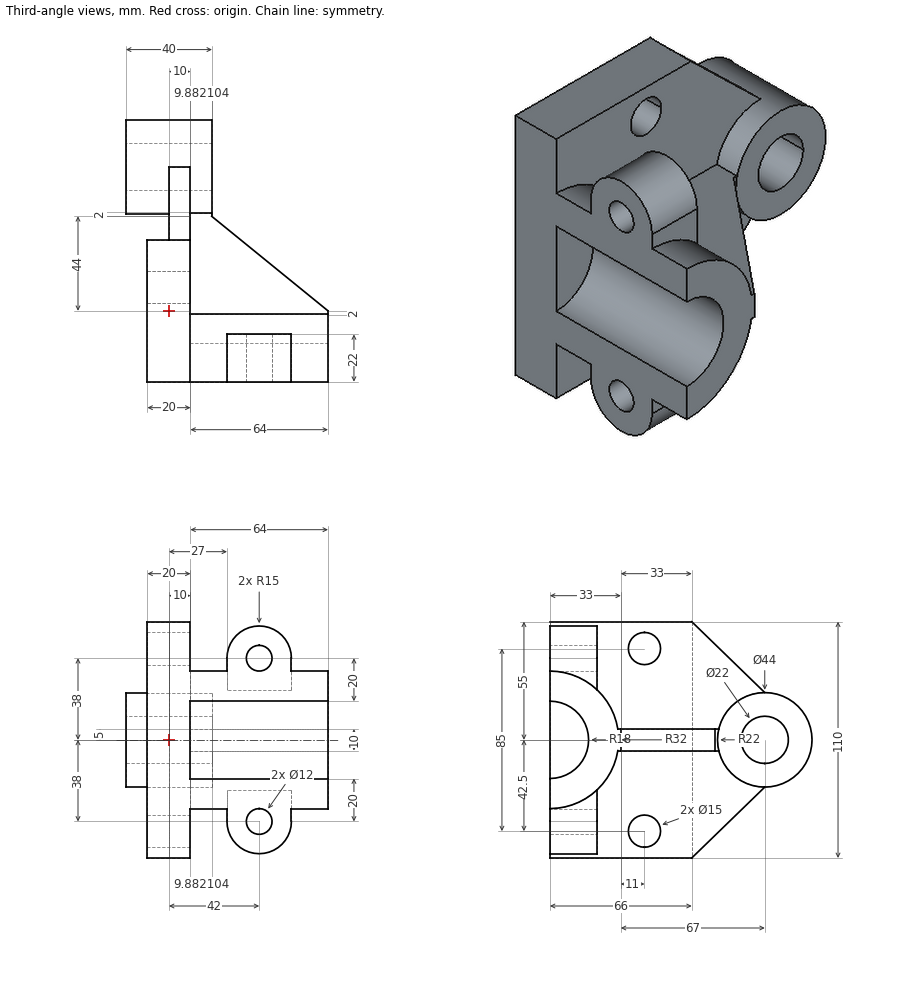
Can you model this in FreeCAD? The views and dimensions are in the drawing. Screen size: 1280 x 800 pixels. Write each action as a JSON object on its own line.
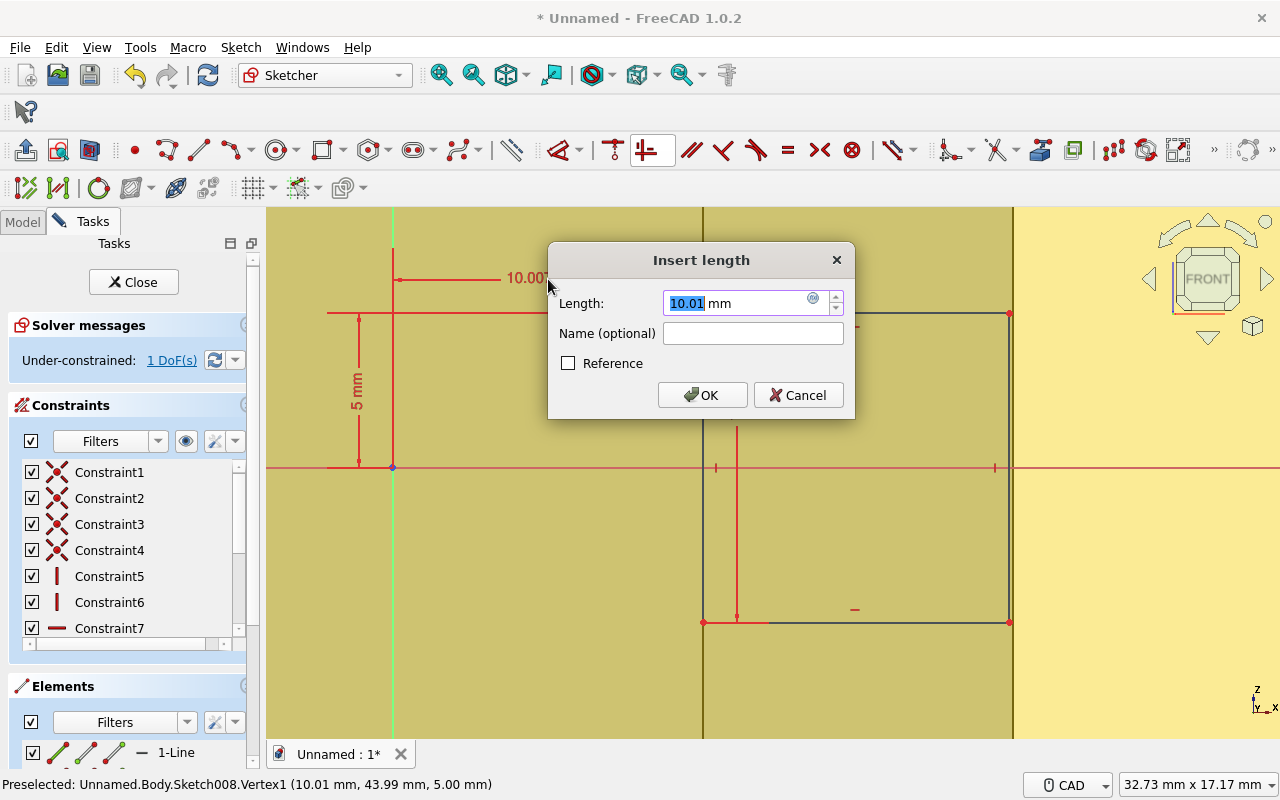
{"action": "type", "text": "10"}
{"action": "key", "text": "Return"}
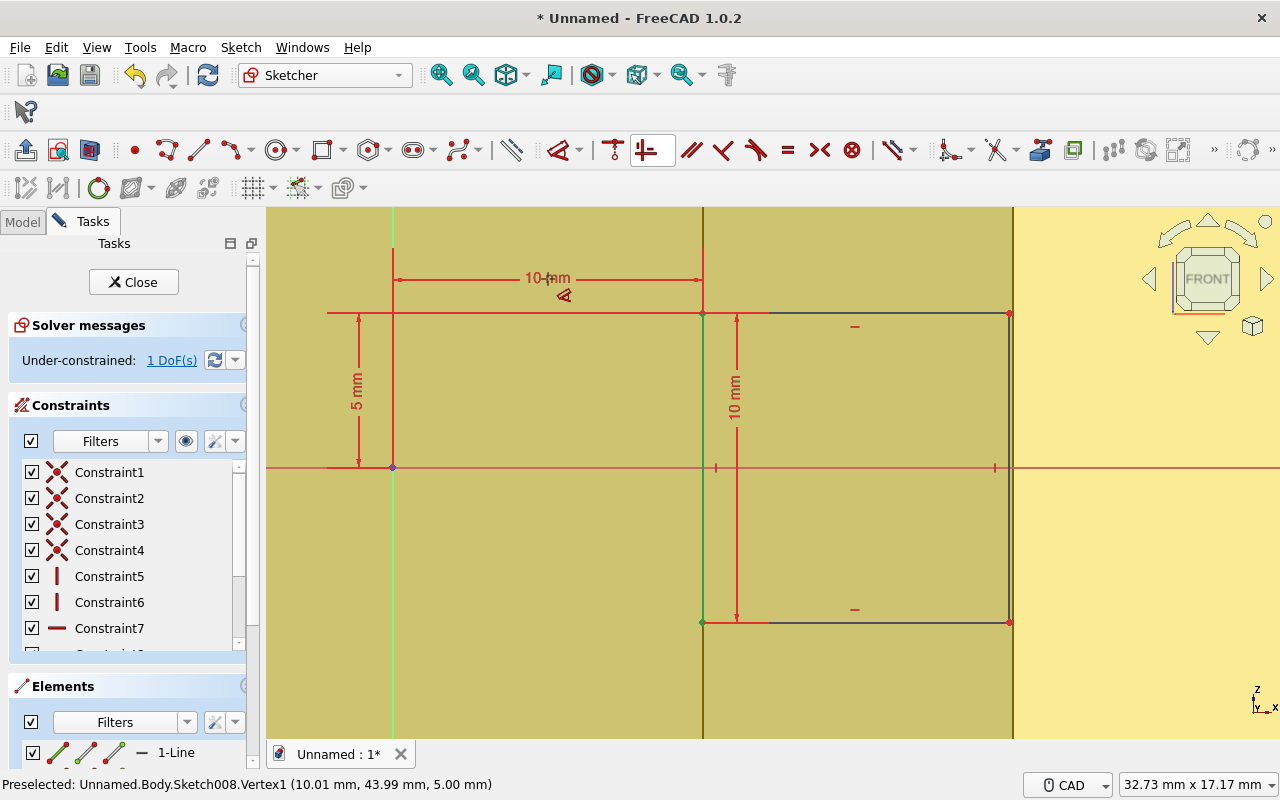
{"action": "left_click", "coordinate": [795, 623]}
{"action": "left_click", "coordinate": [856, 657]}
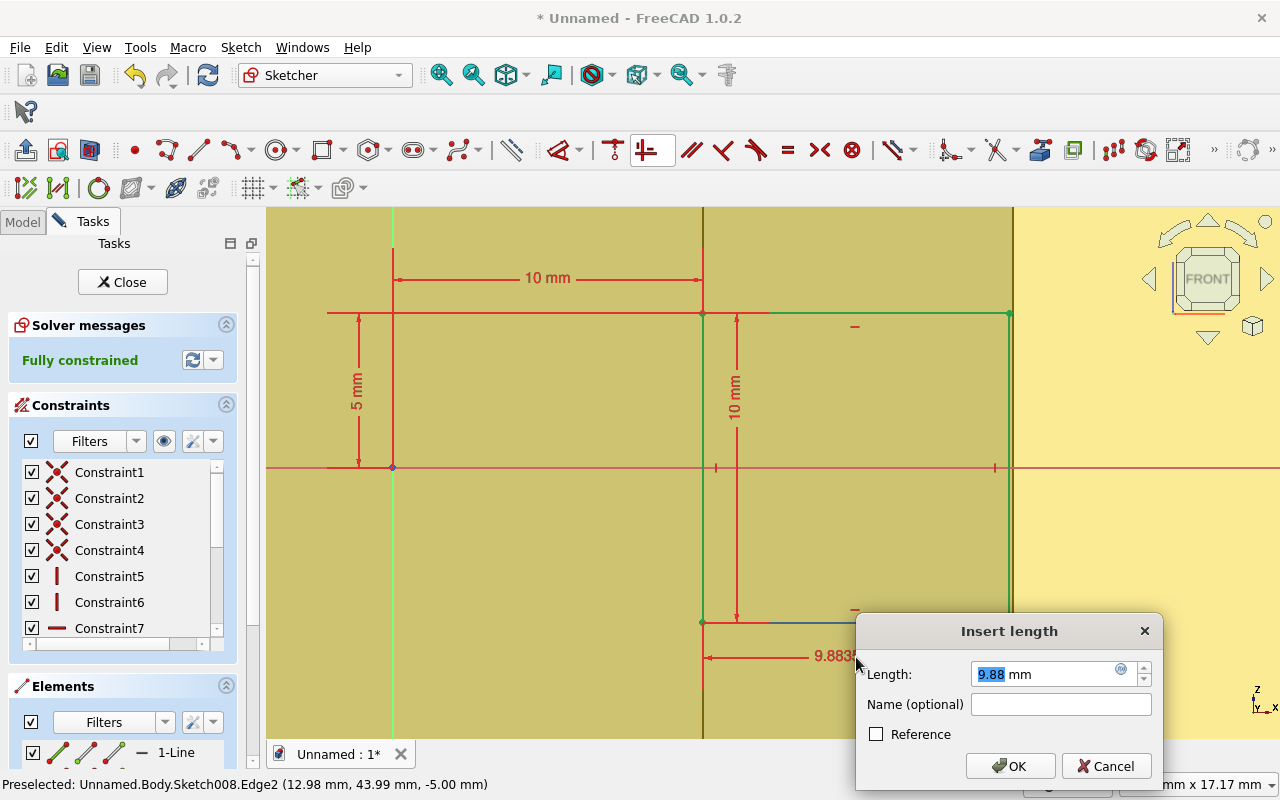
{"action": "type", "text": "9.882104"}
{"action": "key", "text": "Return"}
{"action": "key", "text": "Escape"}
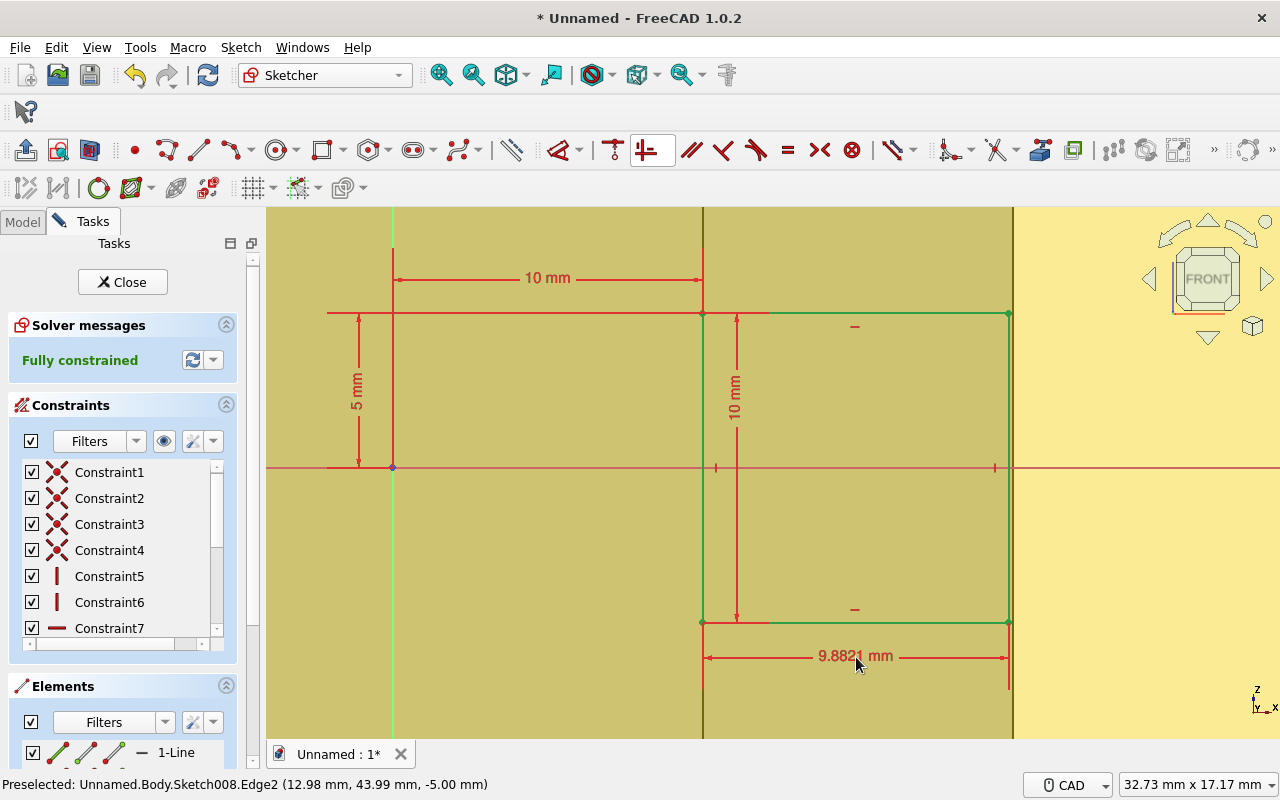
{"action": "left_click", "coordinate": [123, 282]}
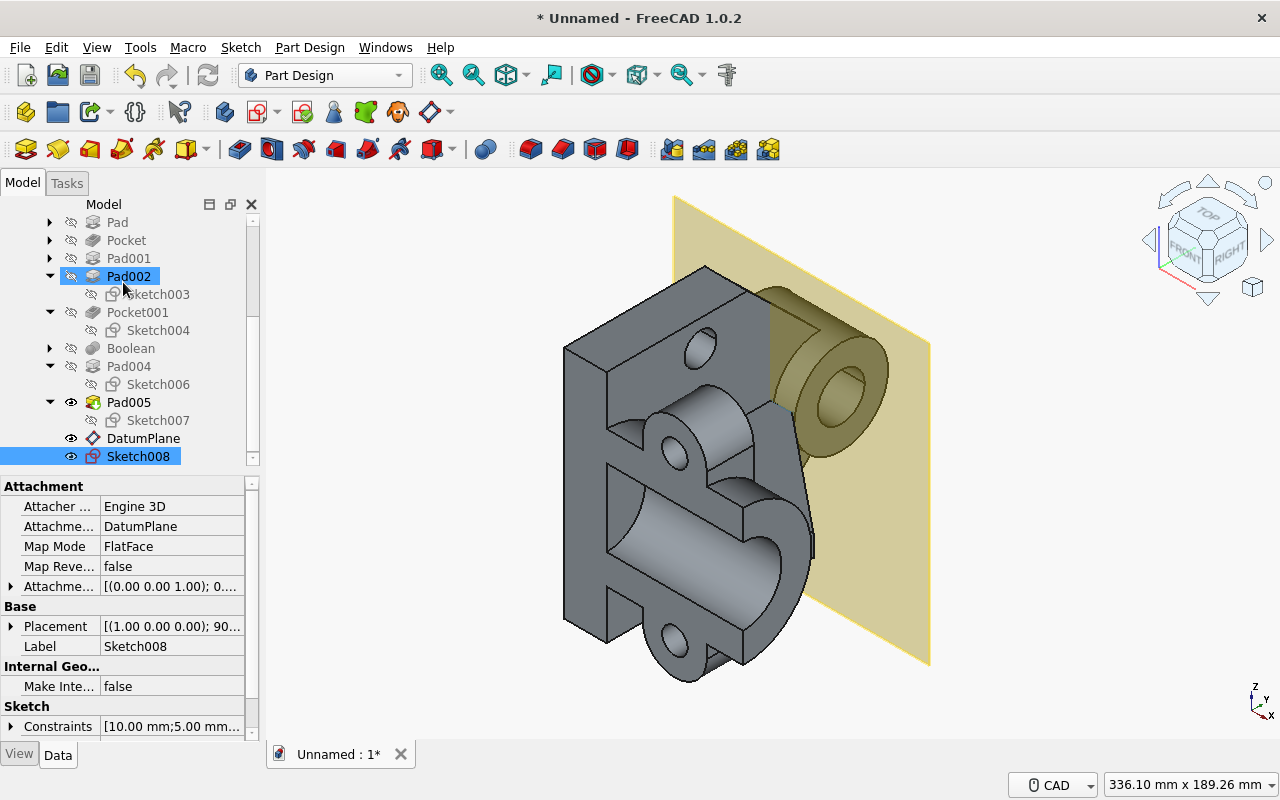
{"action": "left_click", "coordinate": [26, 150]}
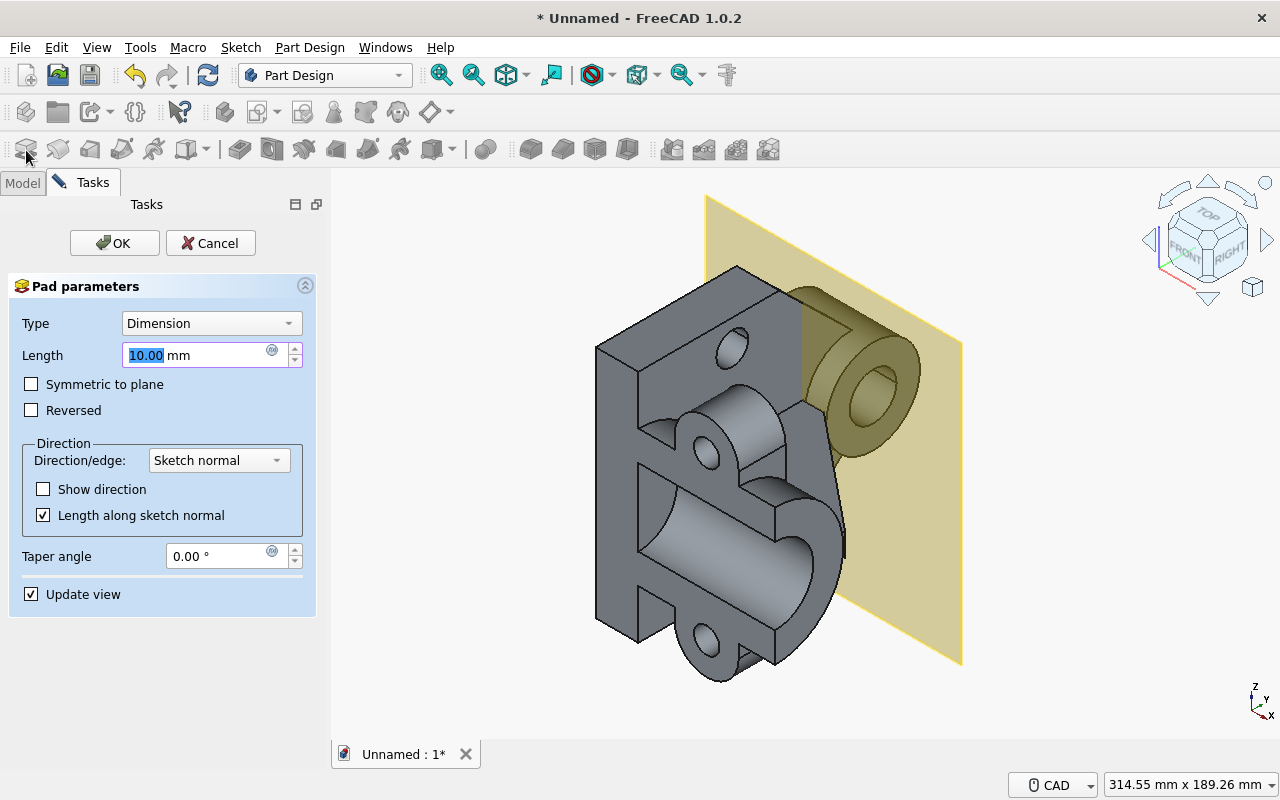
{"action": "type", "text": "2"}
{"action": "key", "text": "Tab"}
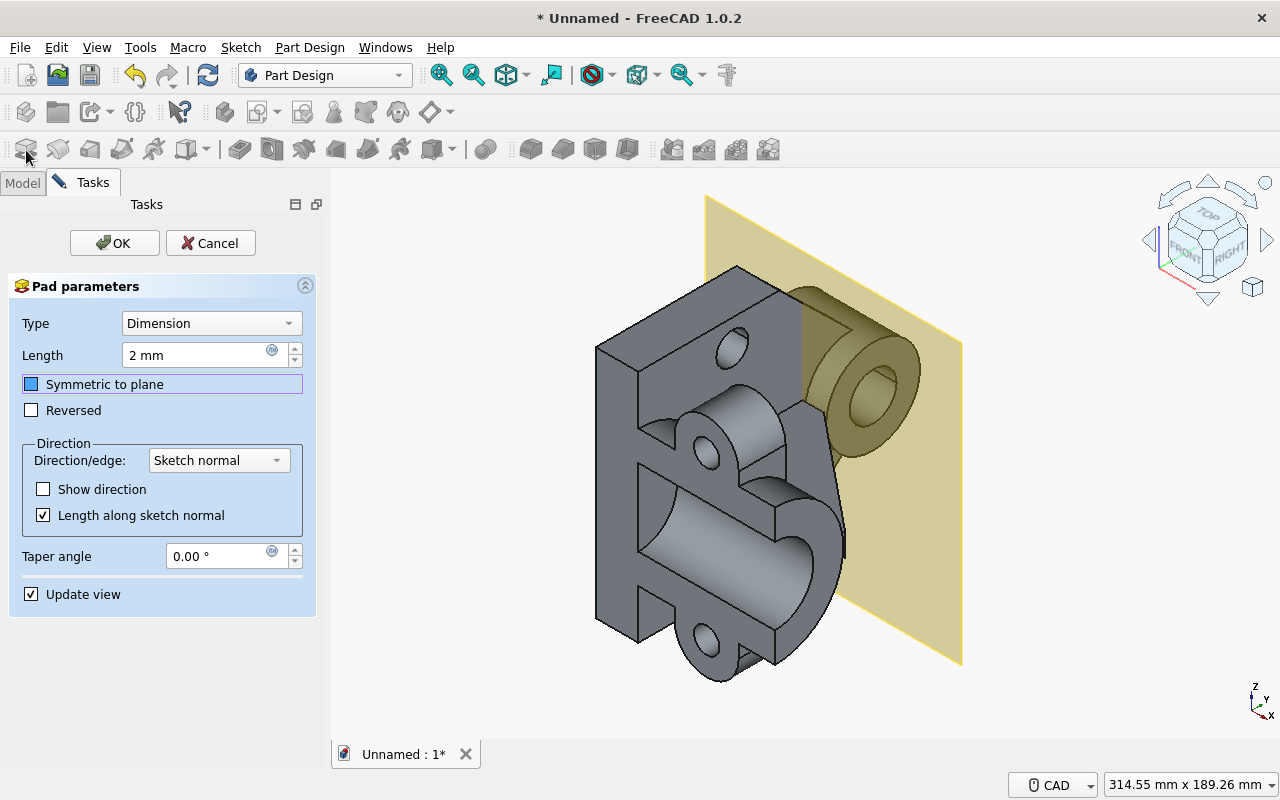
{"action": "left_click", "coordinate": [30, 410]}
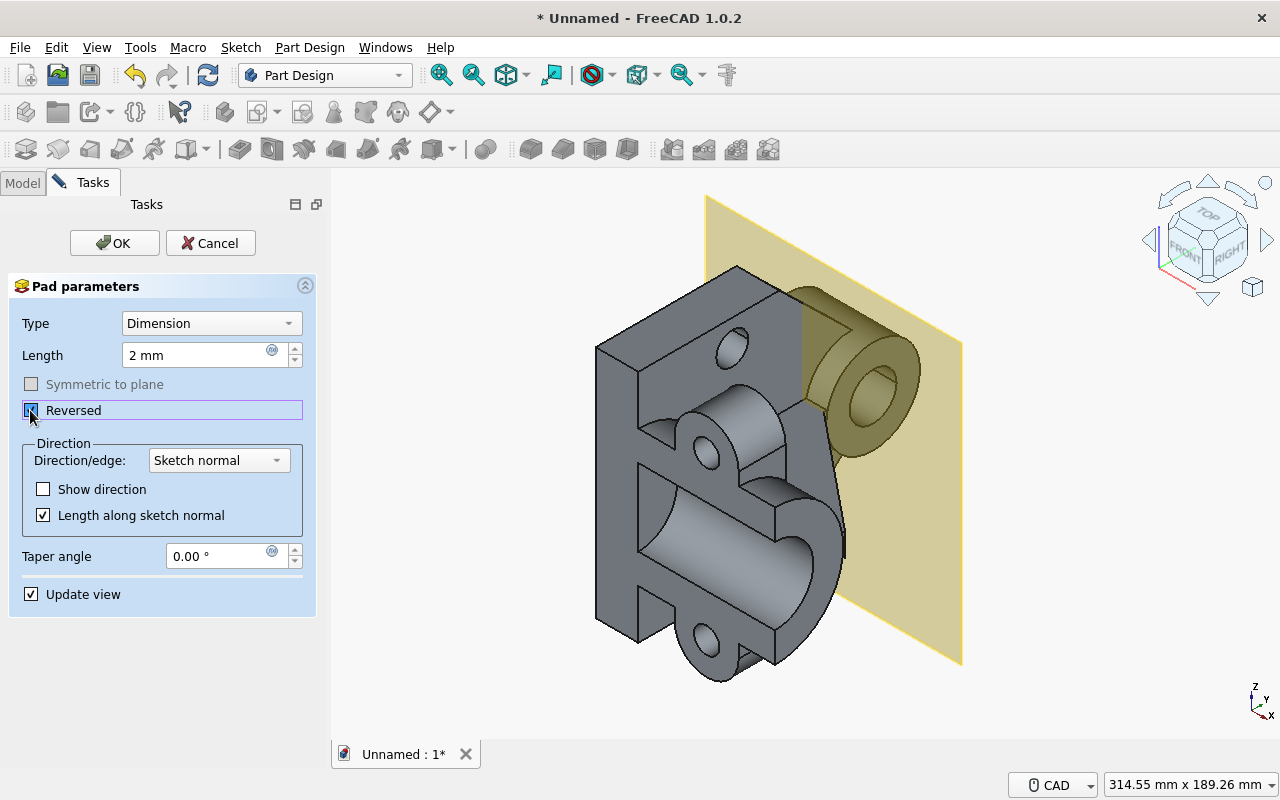
{"action": "left_click", "coordinate": [115, 243]}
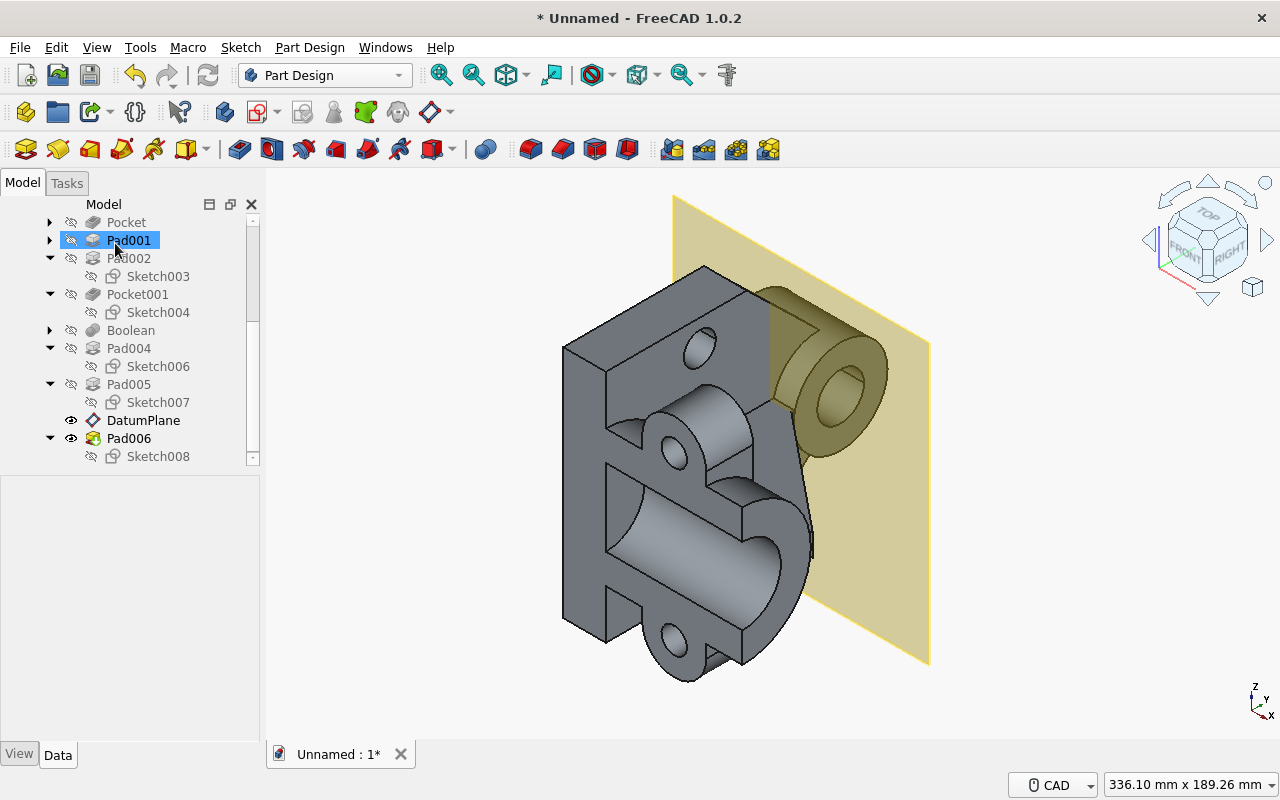
{"action": "left_click", "coordinate": [116, 420]}
{"action": "key", "text": "space"}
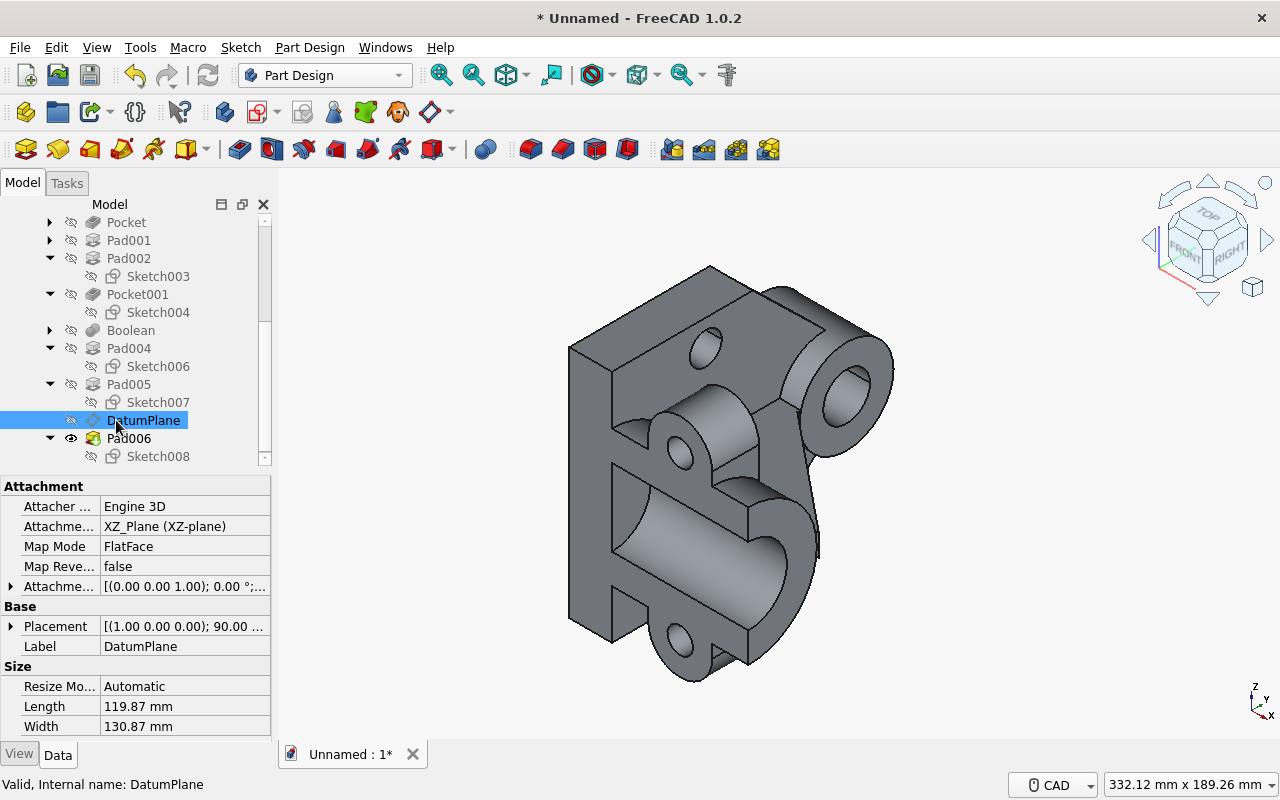
{"action": "left_click", "coordinate": [318, 699]}